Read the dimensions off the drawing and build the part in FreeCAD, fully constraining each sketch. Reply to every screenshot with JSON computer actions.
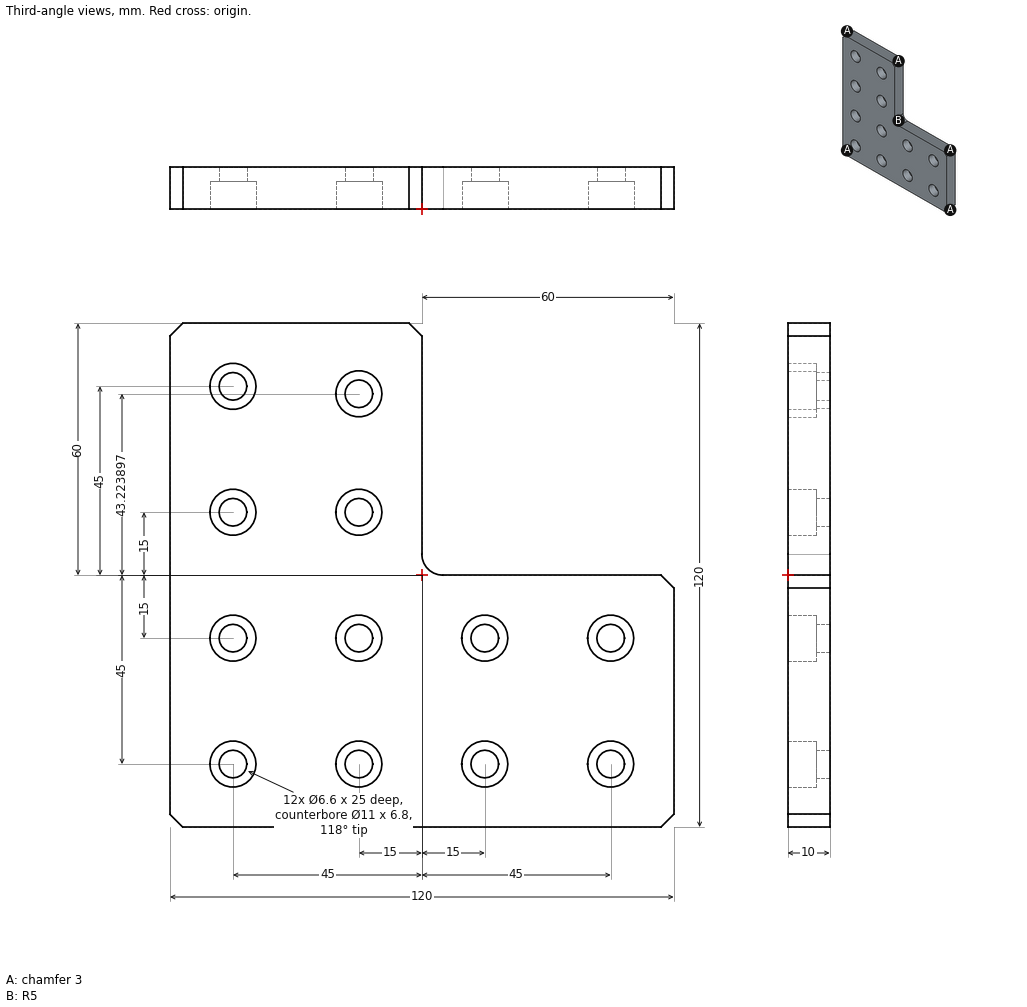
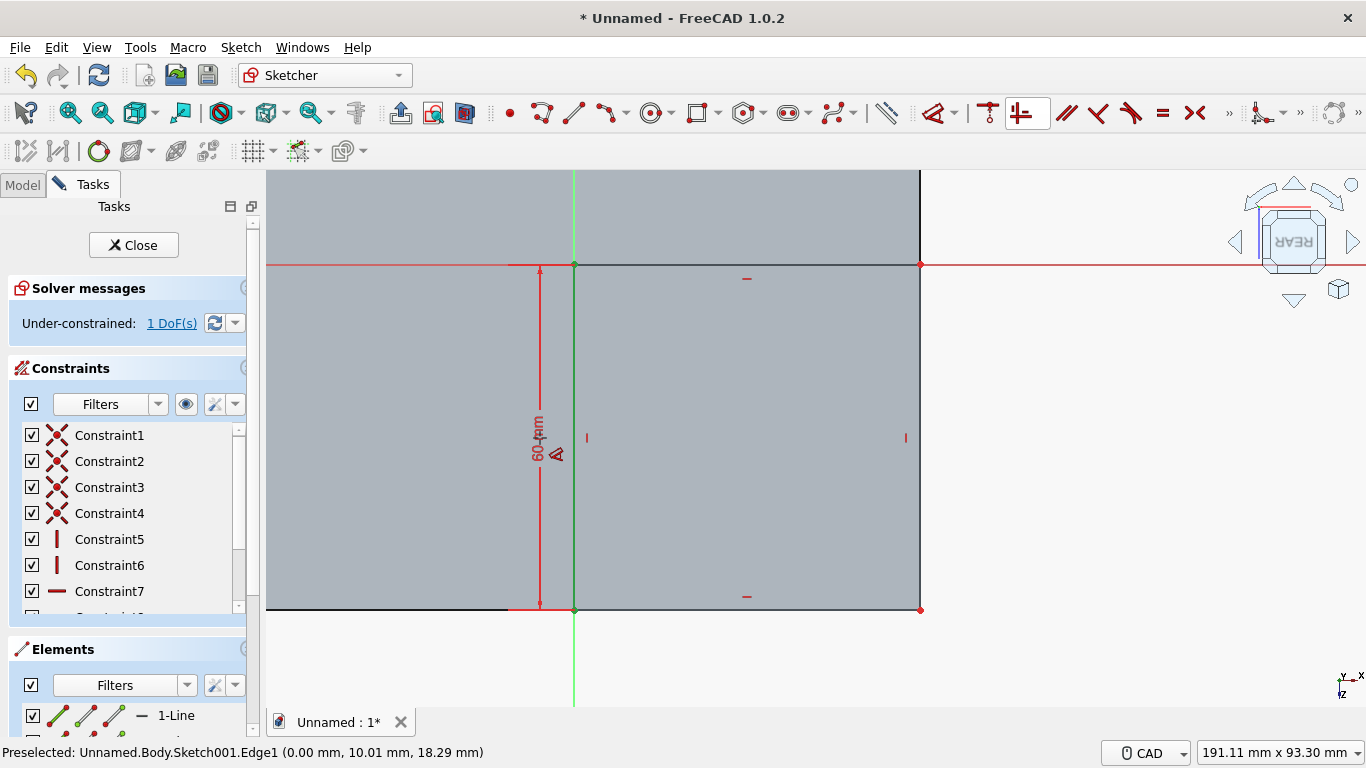
{"action": "left_click", "coordinate": [678, 610]}
{"action": "left_click", "coordinate": [747, 644]}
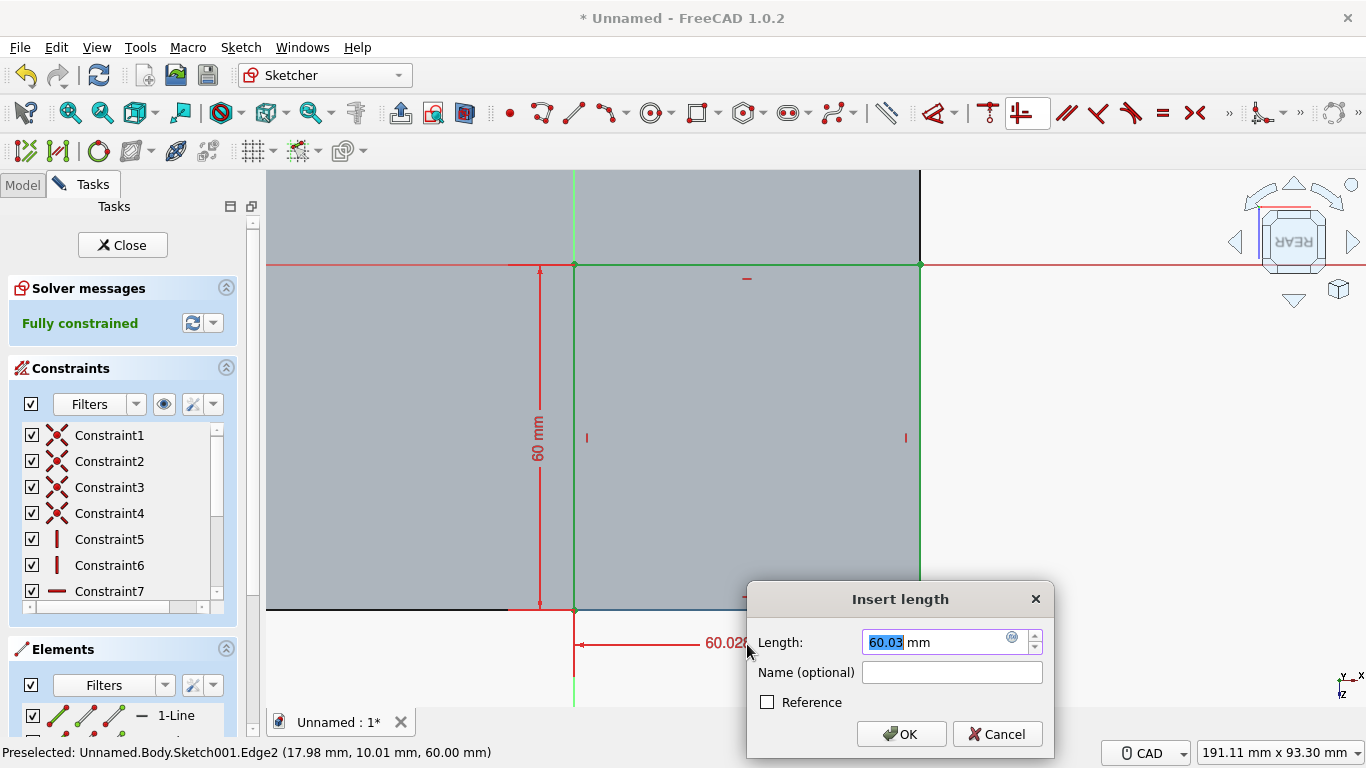
{"action": "type", "text": "60"}
{"action": "key", "text": "Return"}
{"action": "key", "text": "Escape"}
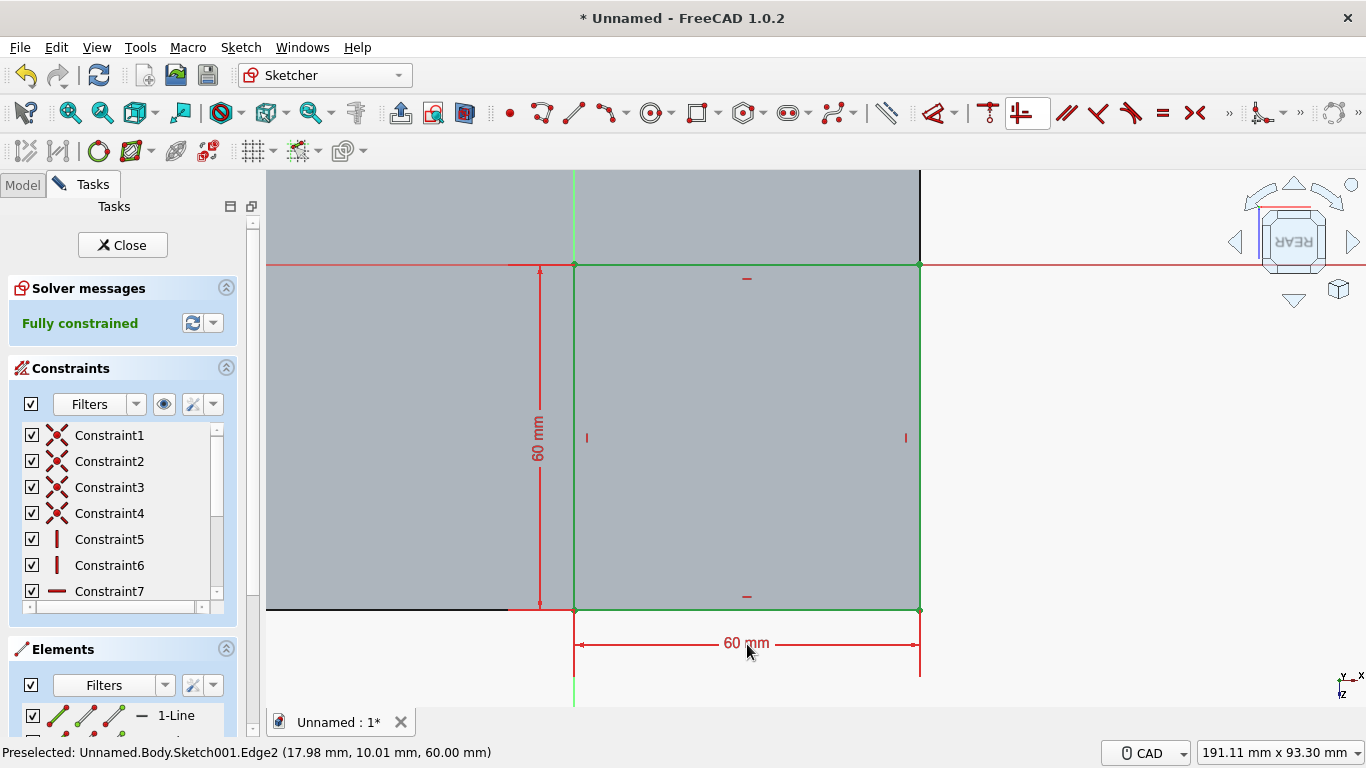
{"action": "left_click", "coordinate": [123, 245]}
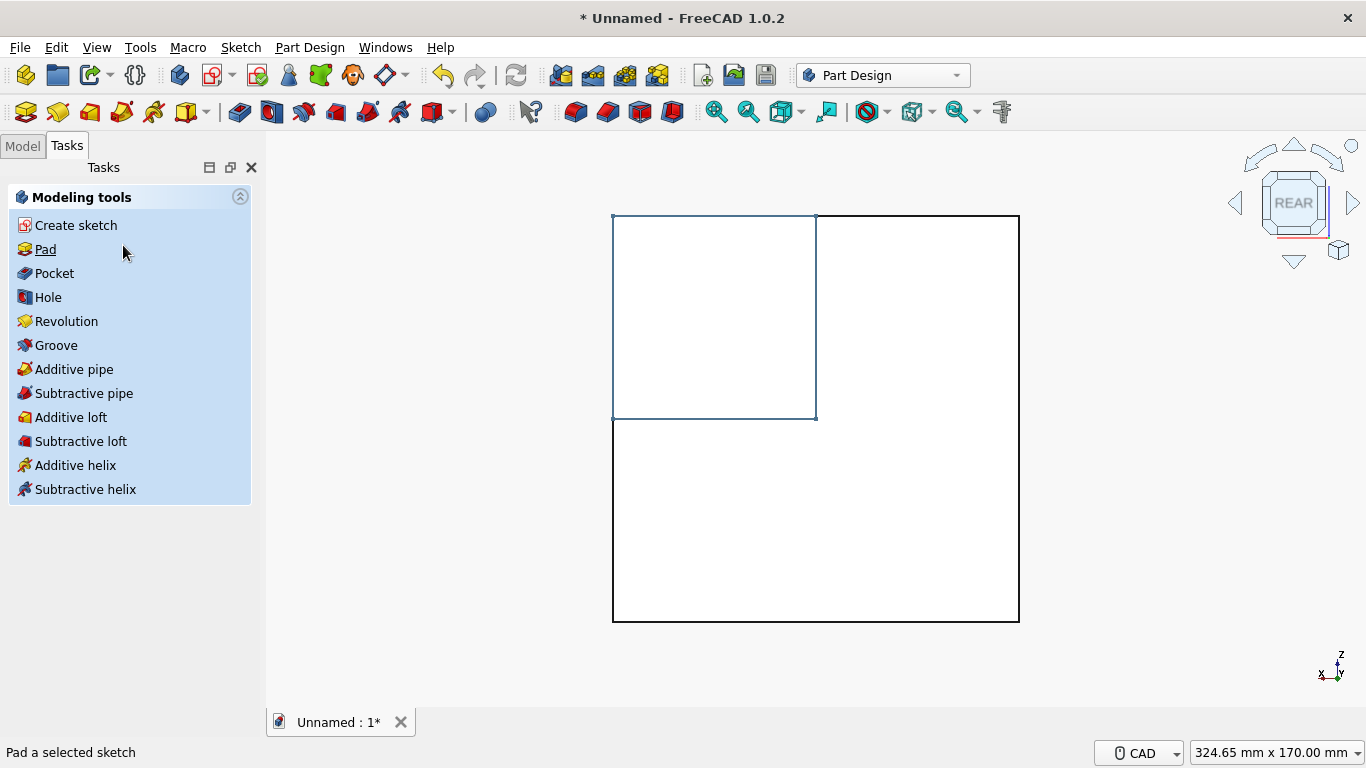
{"action": "left_click", "coordinate": [240, 112]}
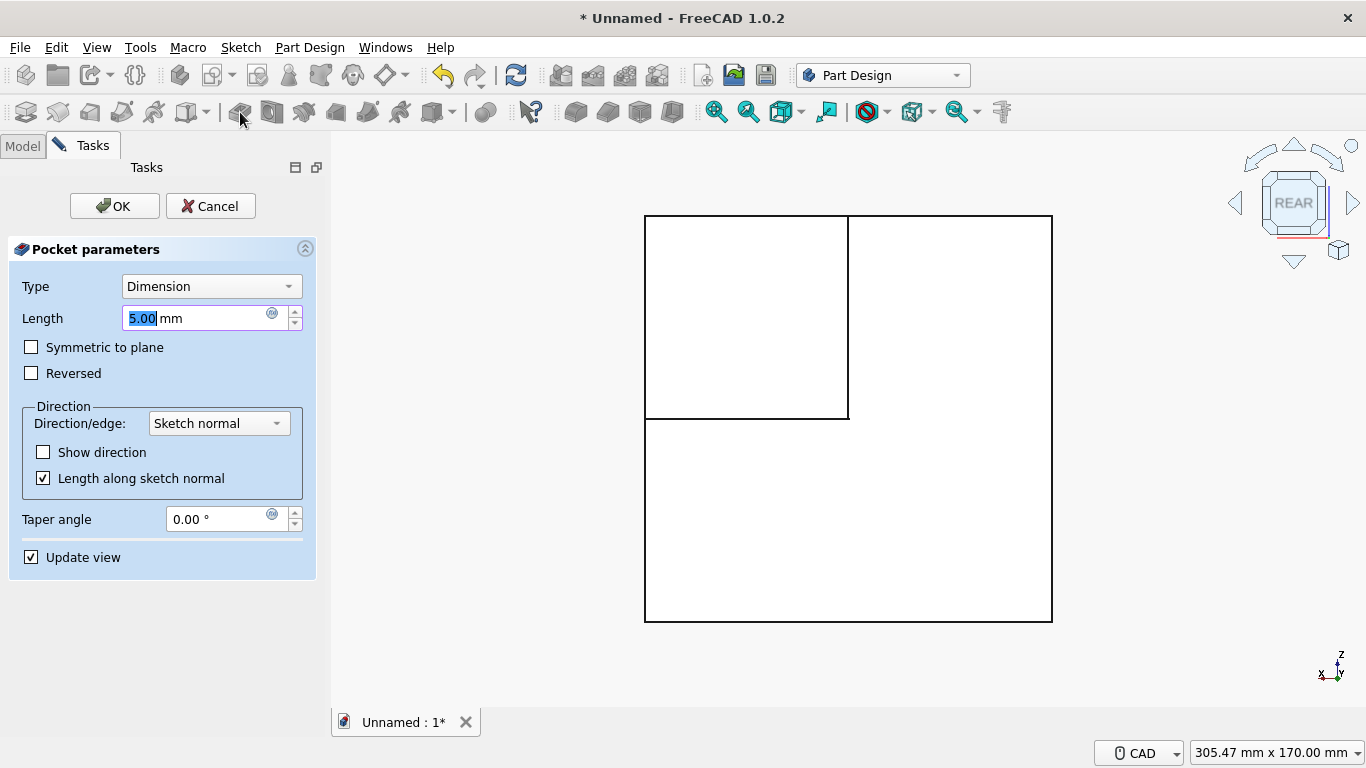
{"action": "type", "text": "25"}
{"action": "key", "text": "Tab"}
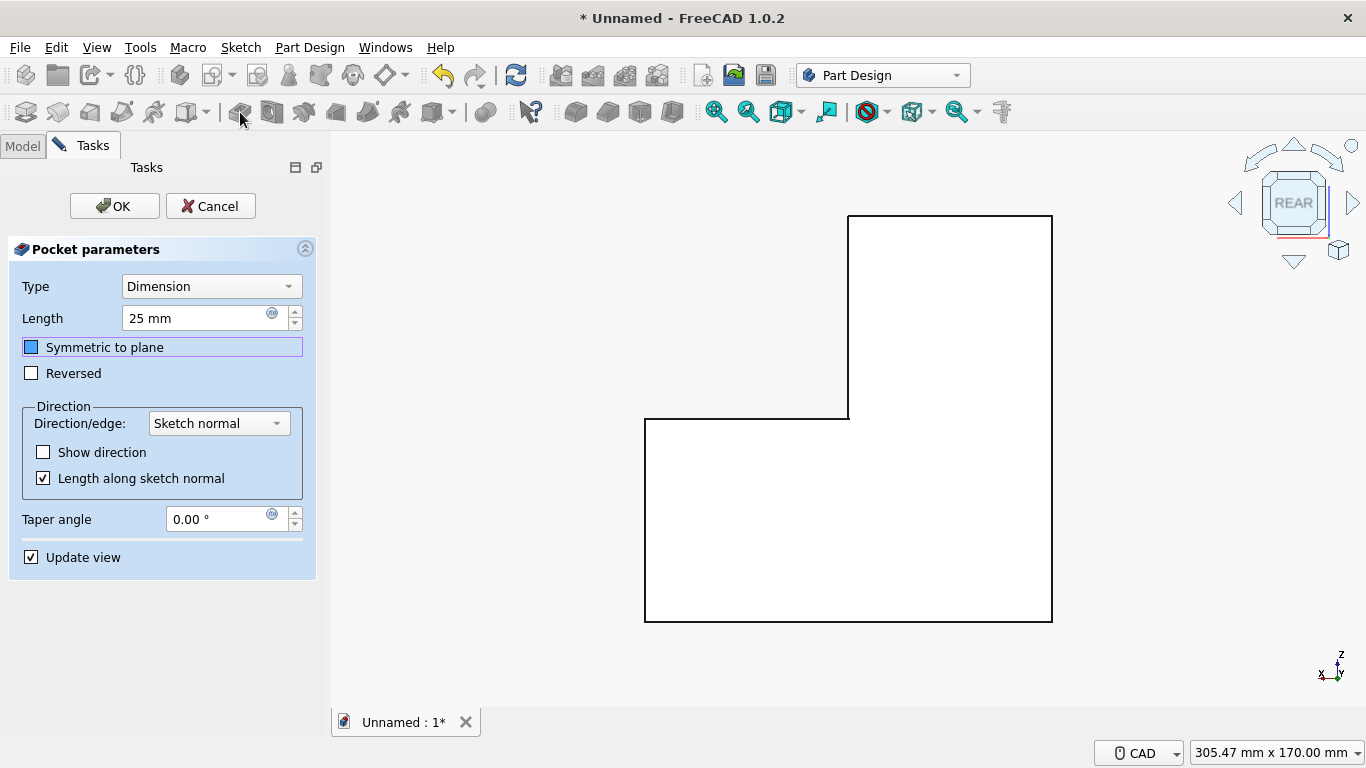
{"action": "left_click", "coordinate": [115, 206]}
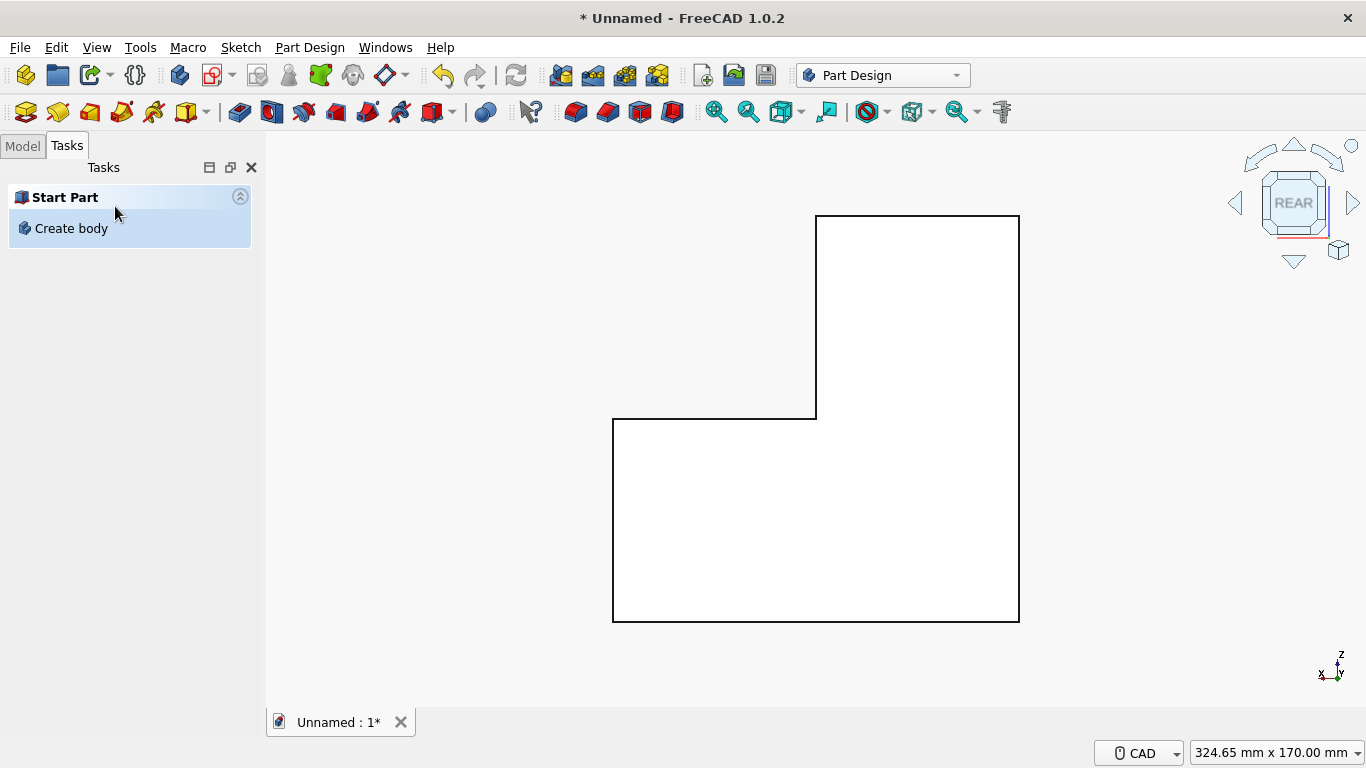
{"action": "key", "text": "0"}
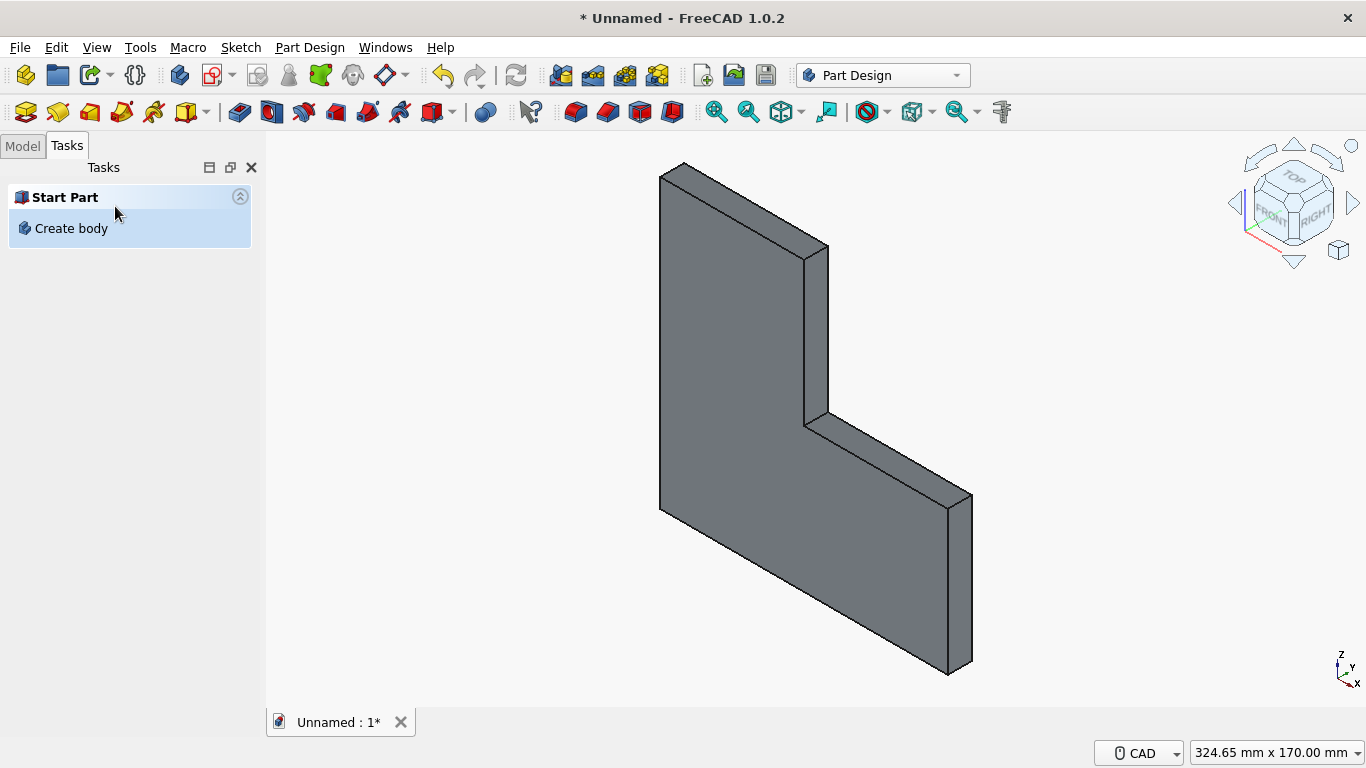
{"action": "left_click", "coordinate": [960, 501]}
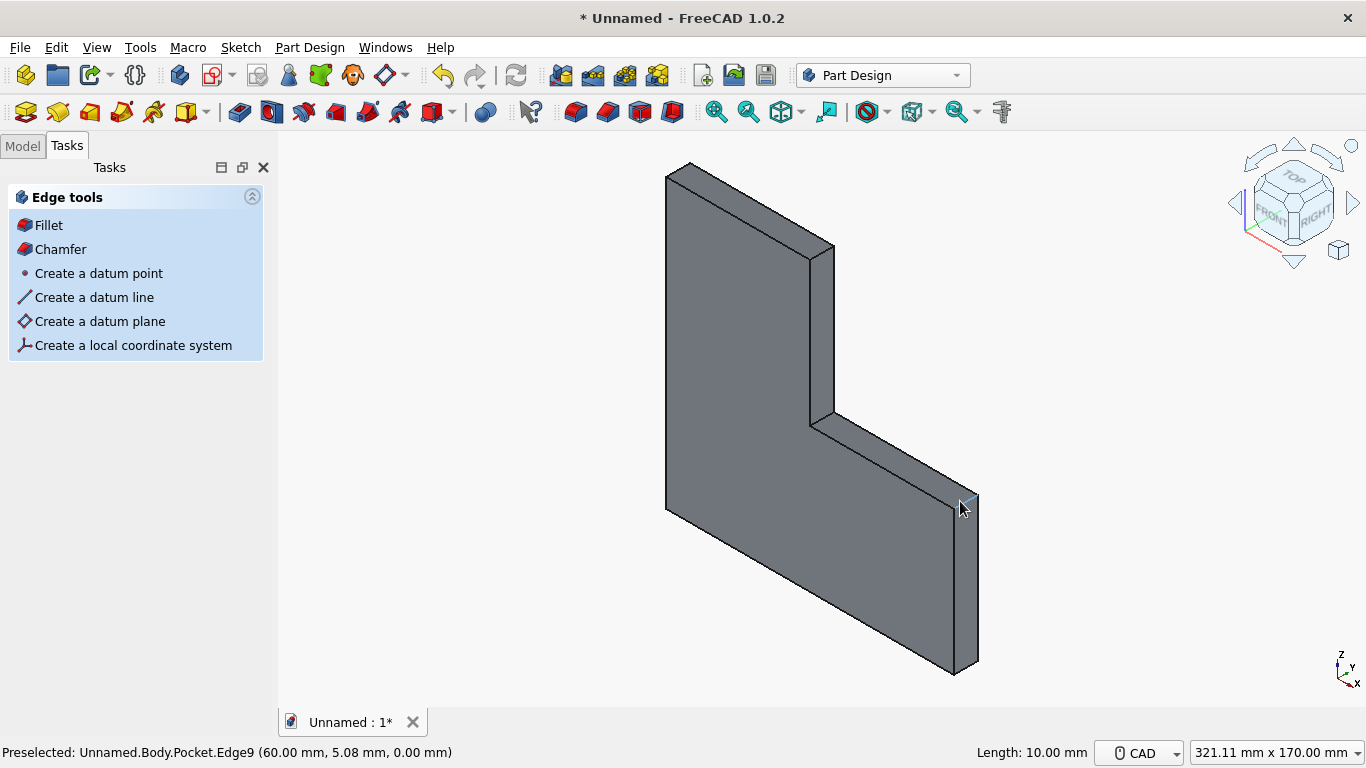
{"action": "left_click", "coordinate": [822, 252], "text": "ctrl"}